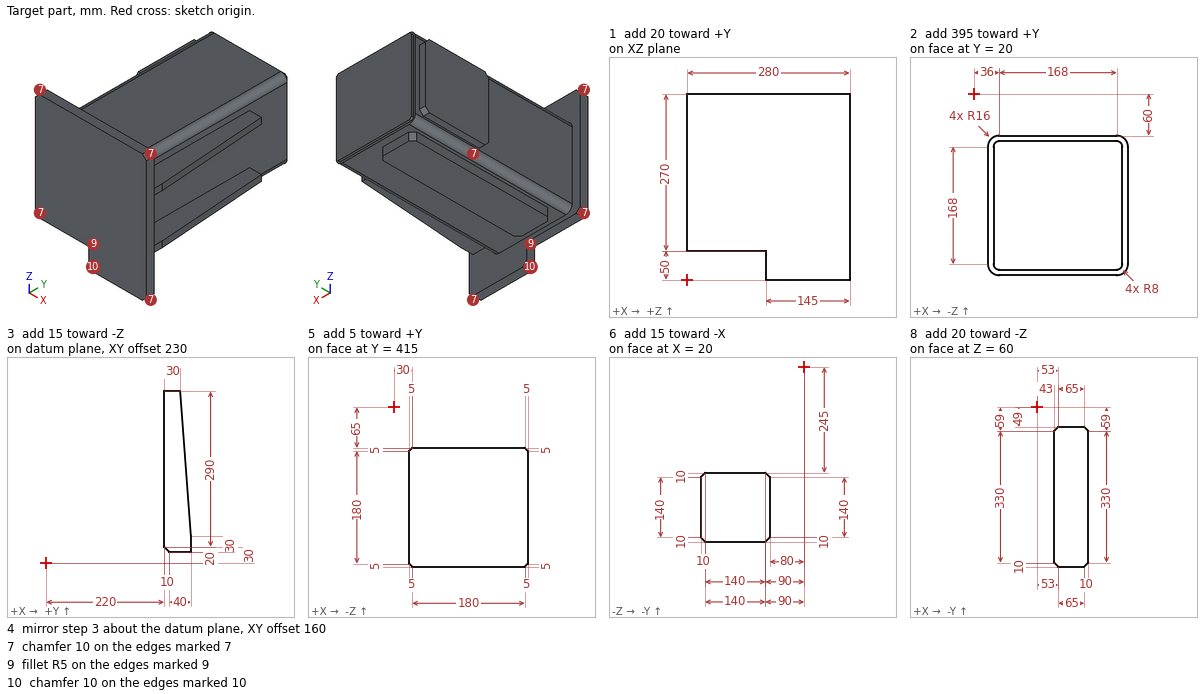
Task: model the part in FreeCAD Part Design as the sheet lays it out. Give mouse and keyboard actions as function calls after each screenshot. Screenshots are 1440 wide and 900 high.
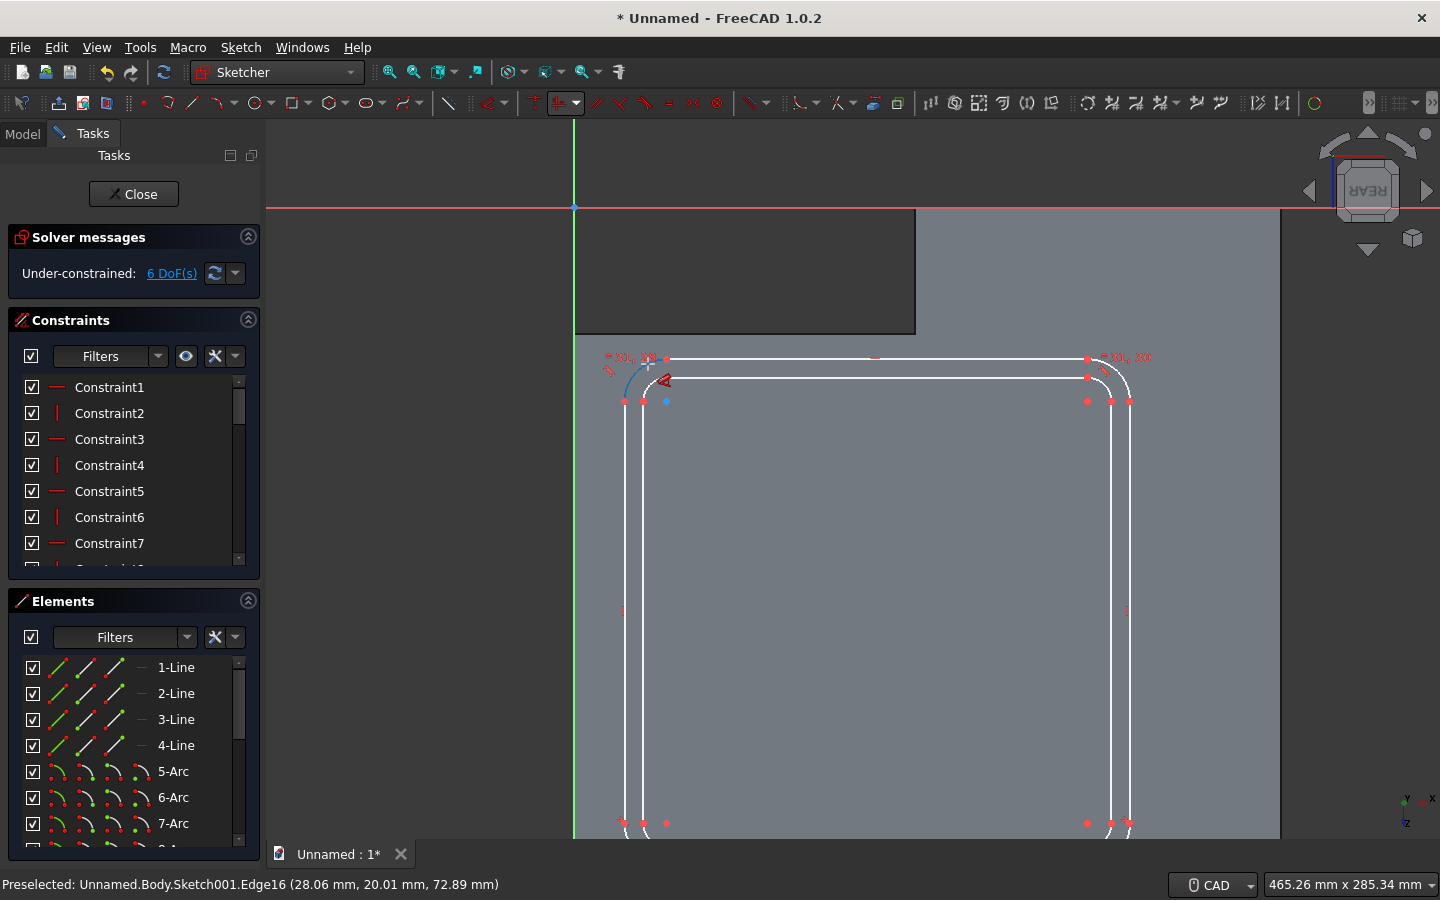
click(648, 364)
click(634, 335)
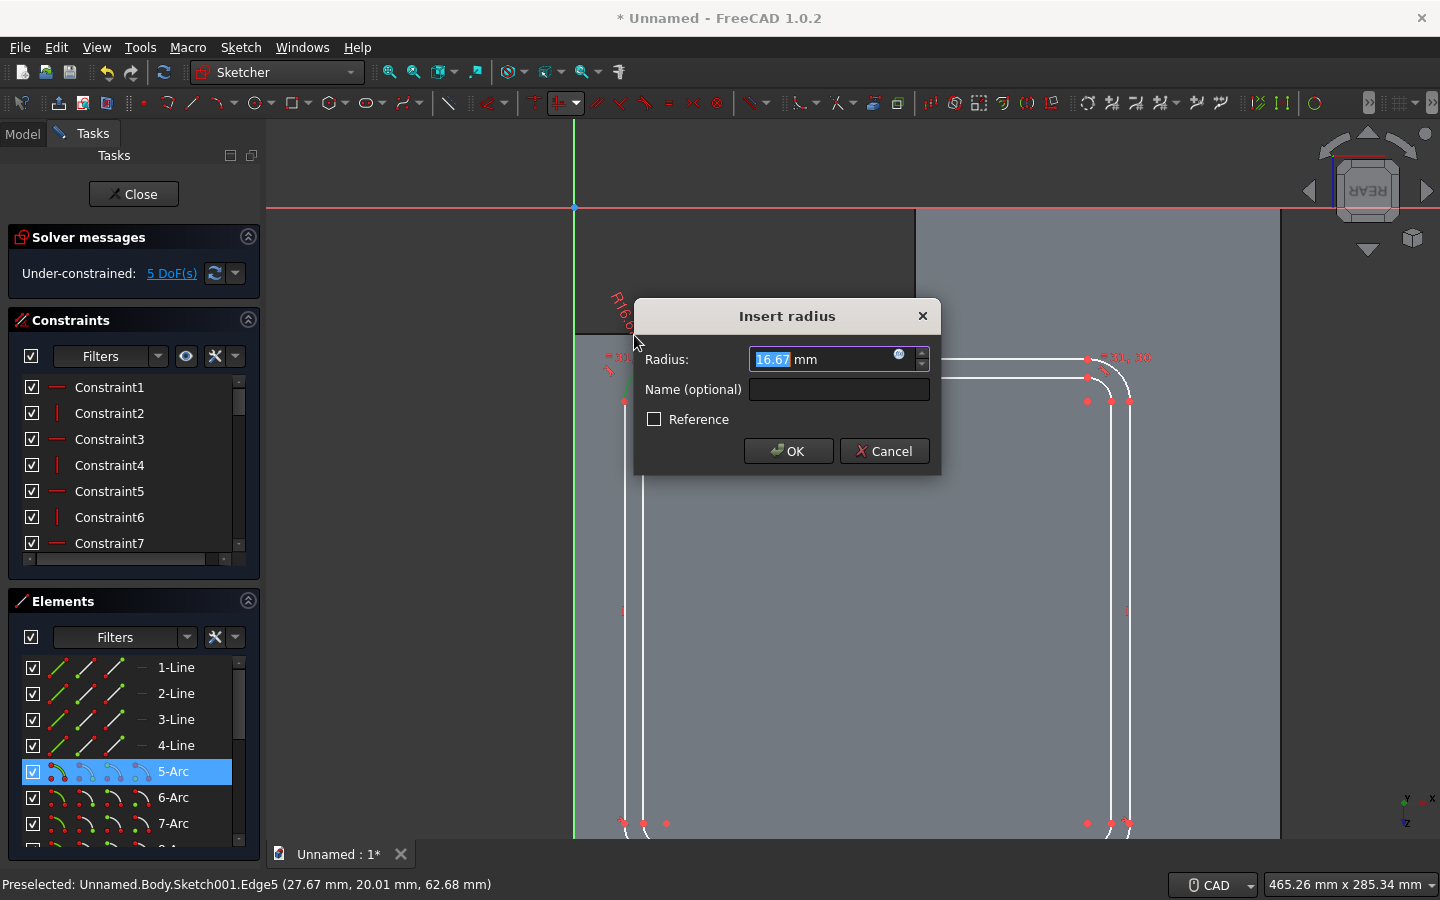
text(16)
key(Return)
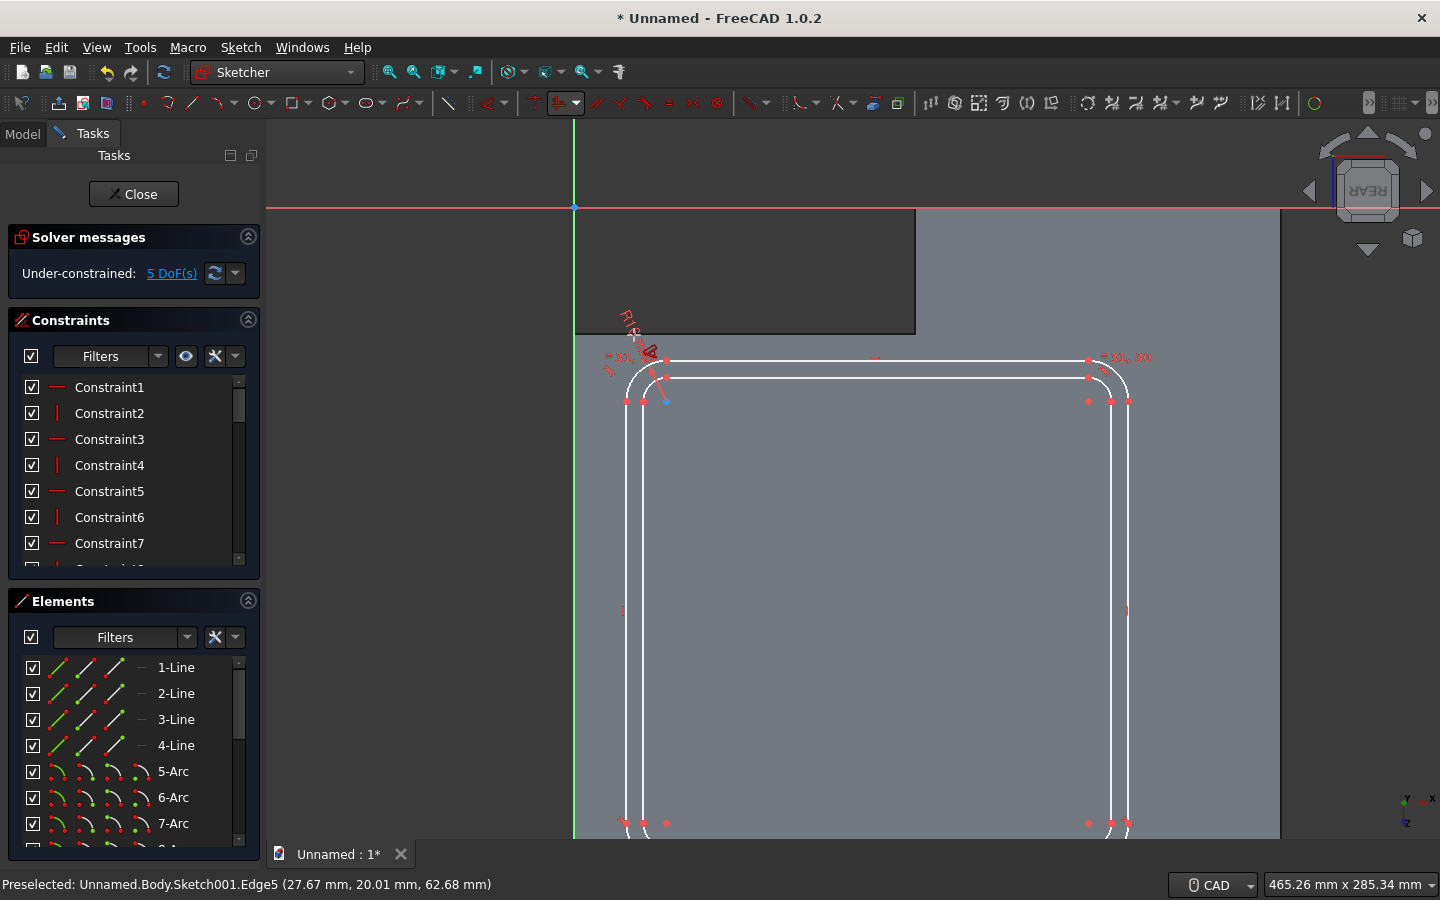
scroll(1109, 391, up, 4)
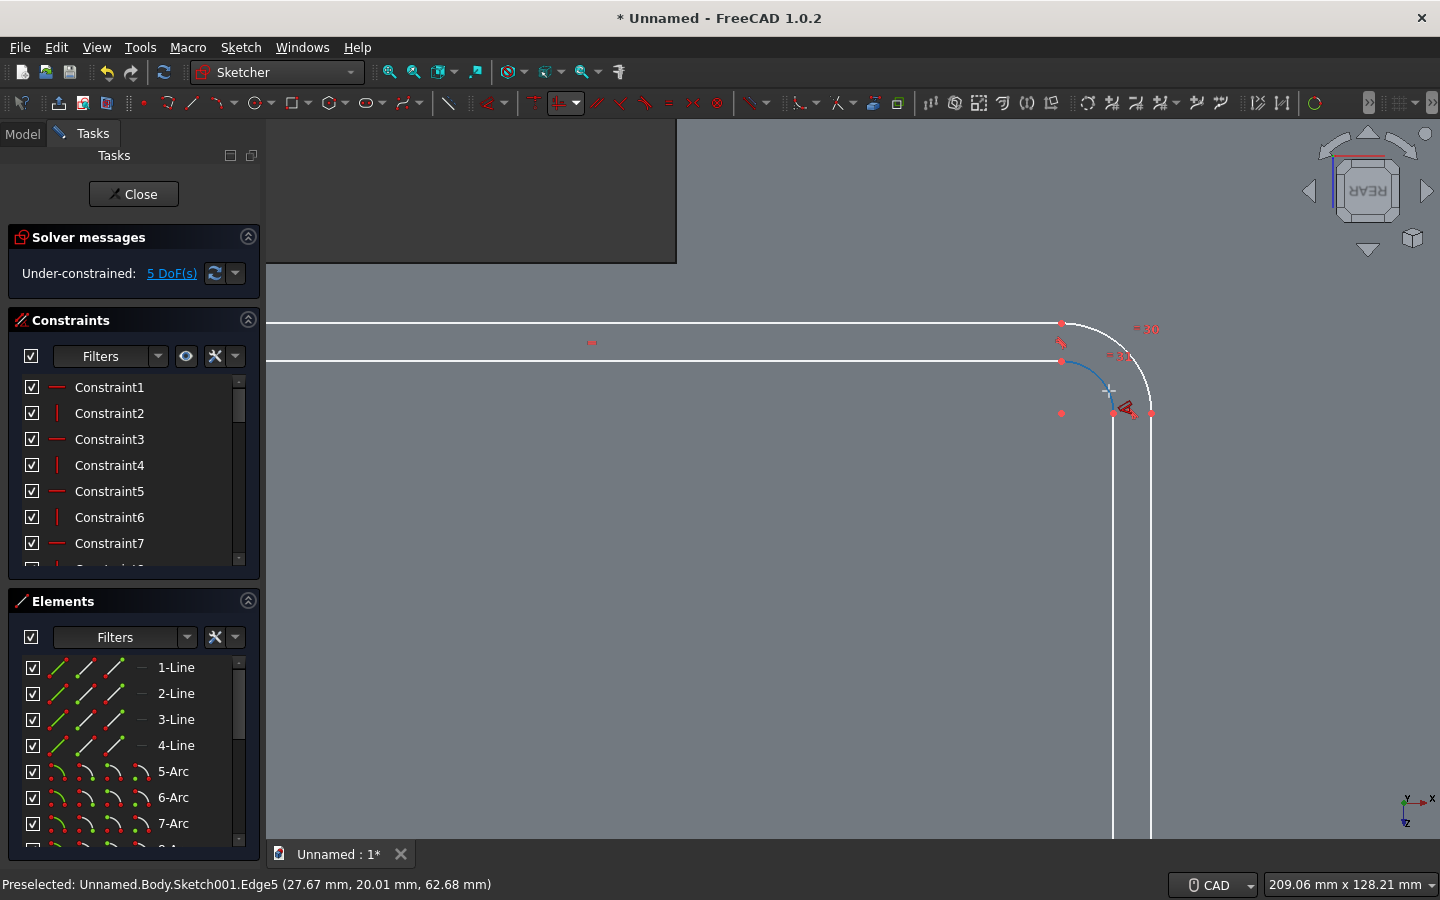
click(1108, 390)
click(1134, 456)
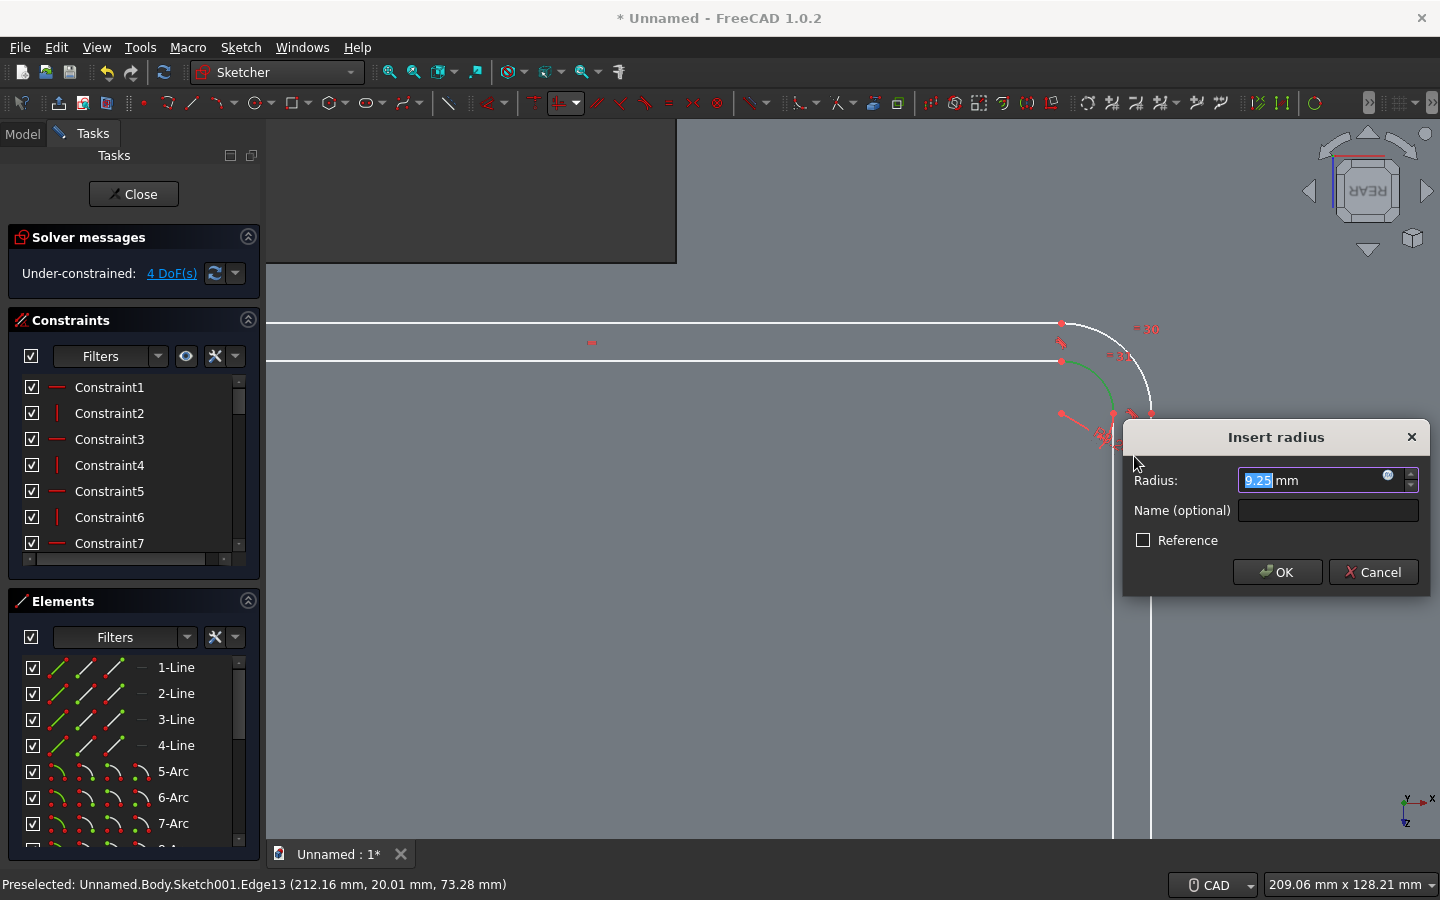
text(8)
key(Return)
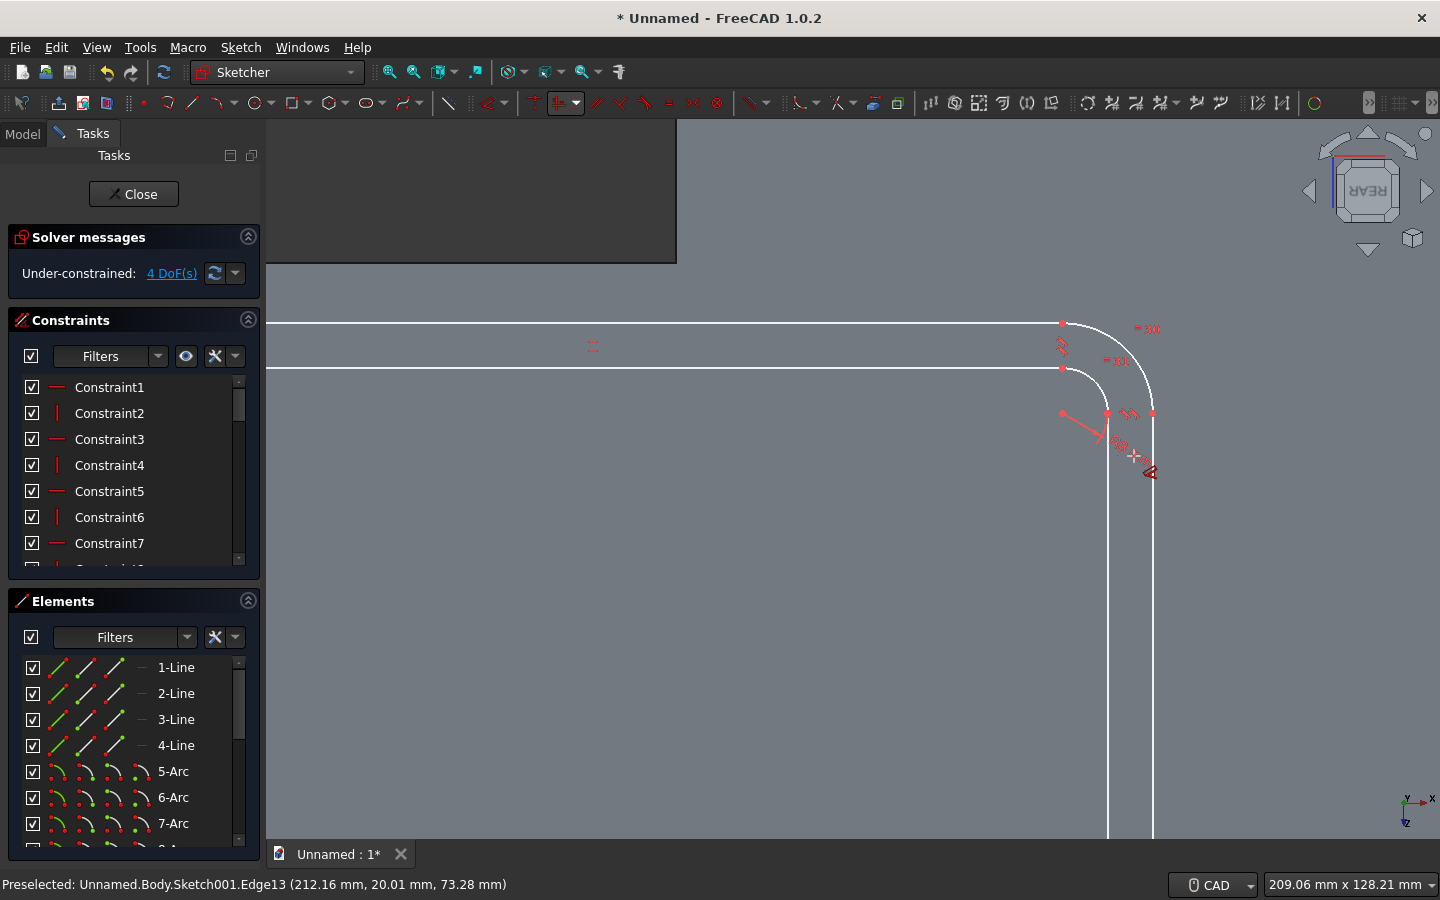
click(781, 323)
click(678, 289)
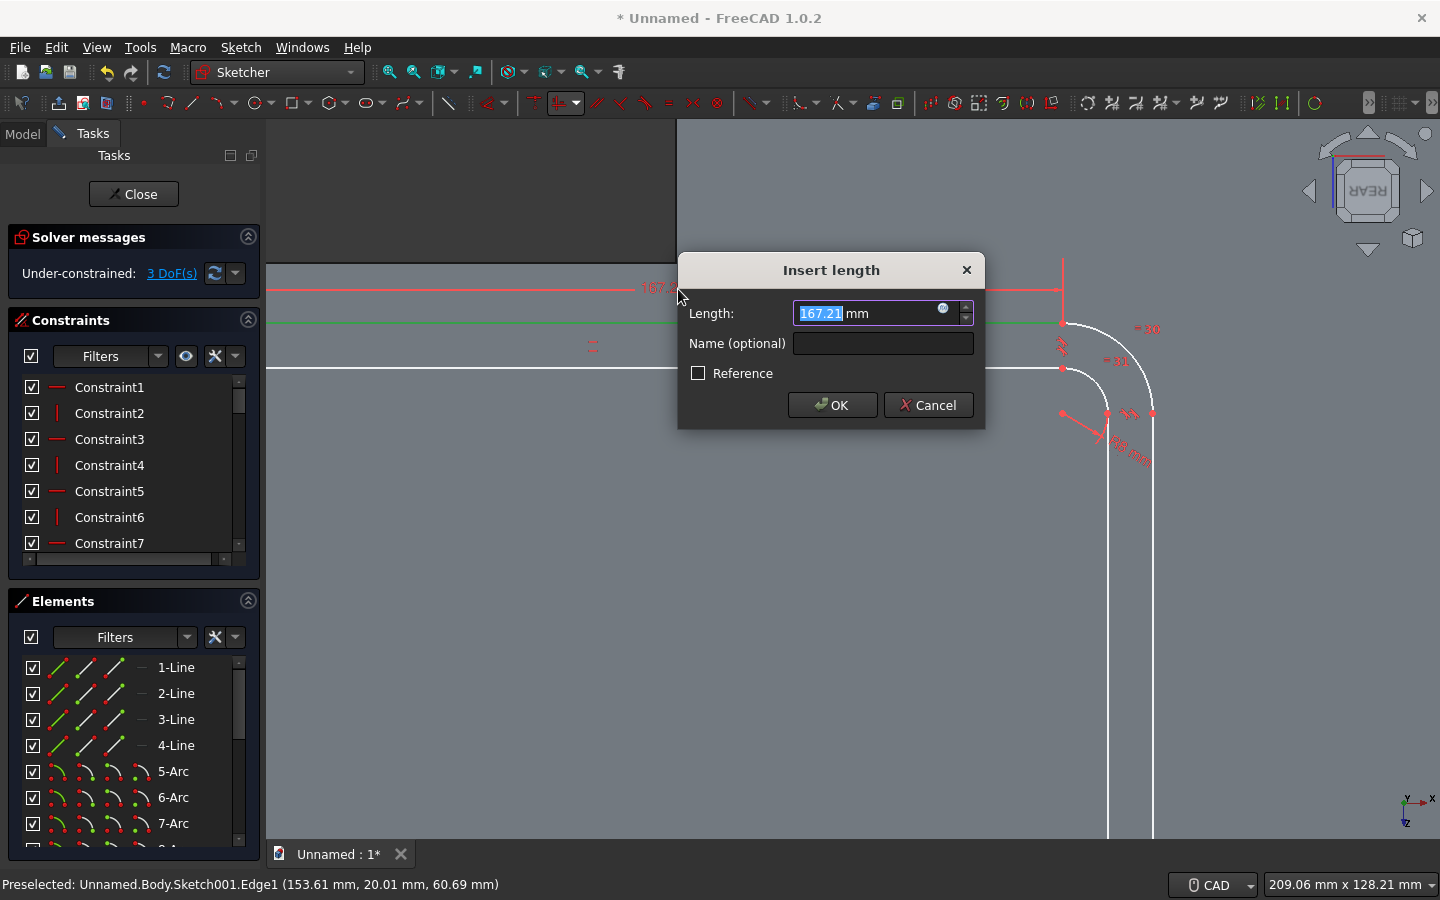
text(168)
key(Return)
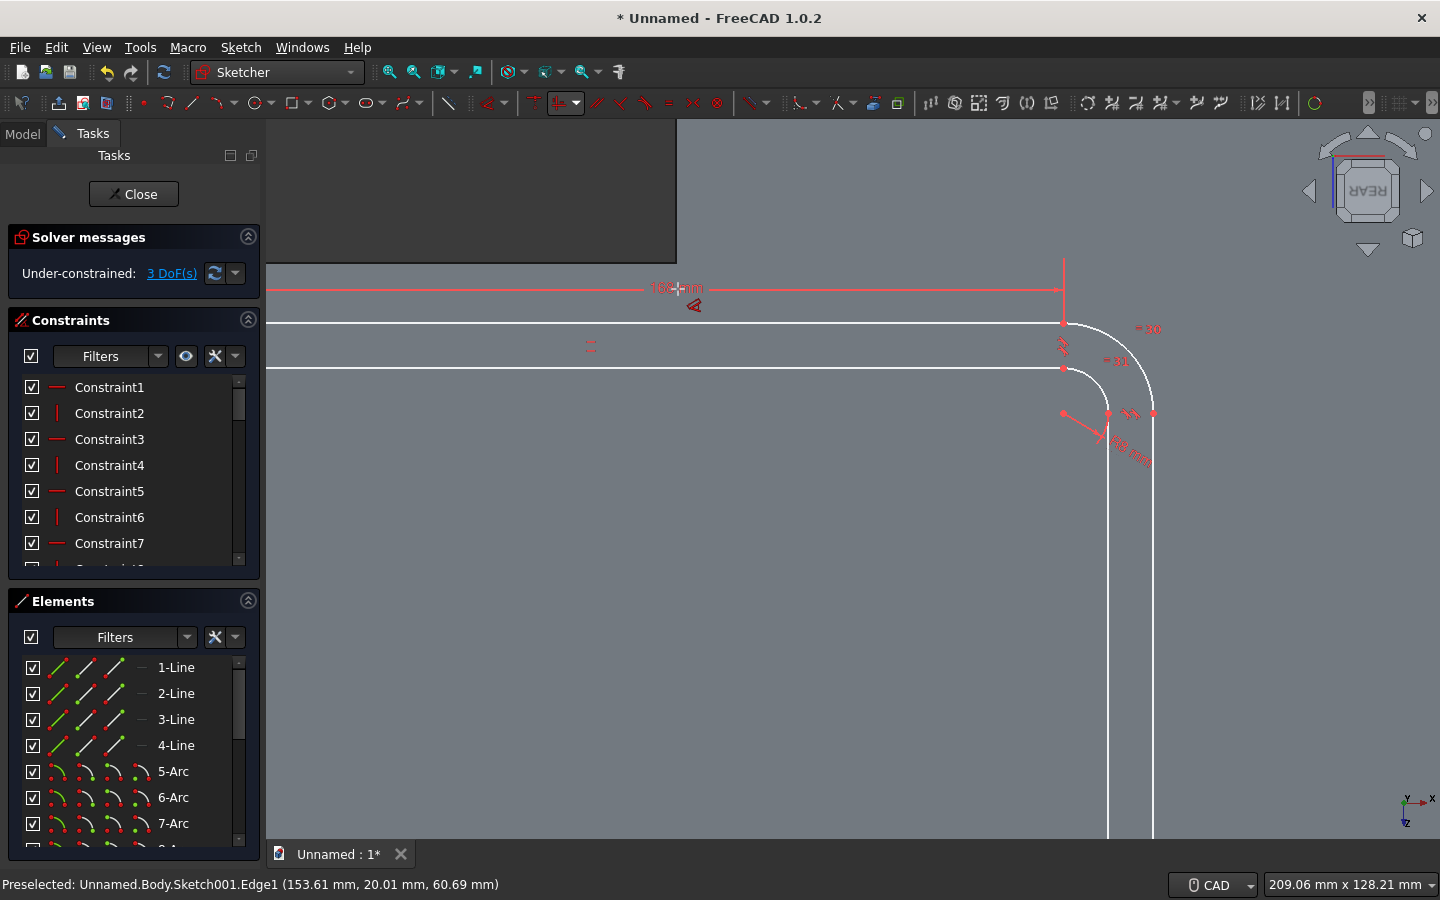
scroll(892, 378, down, 6)